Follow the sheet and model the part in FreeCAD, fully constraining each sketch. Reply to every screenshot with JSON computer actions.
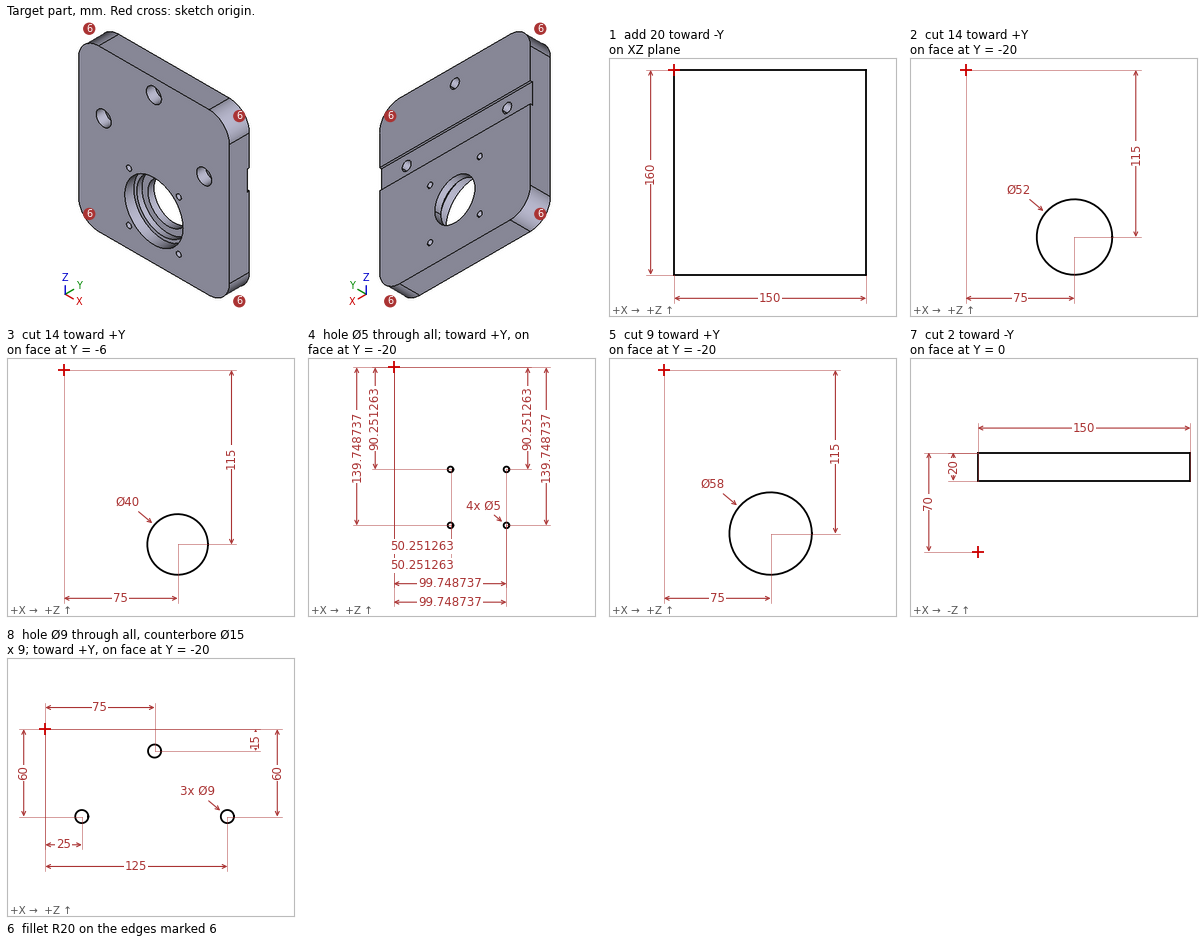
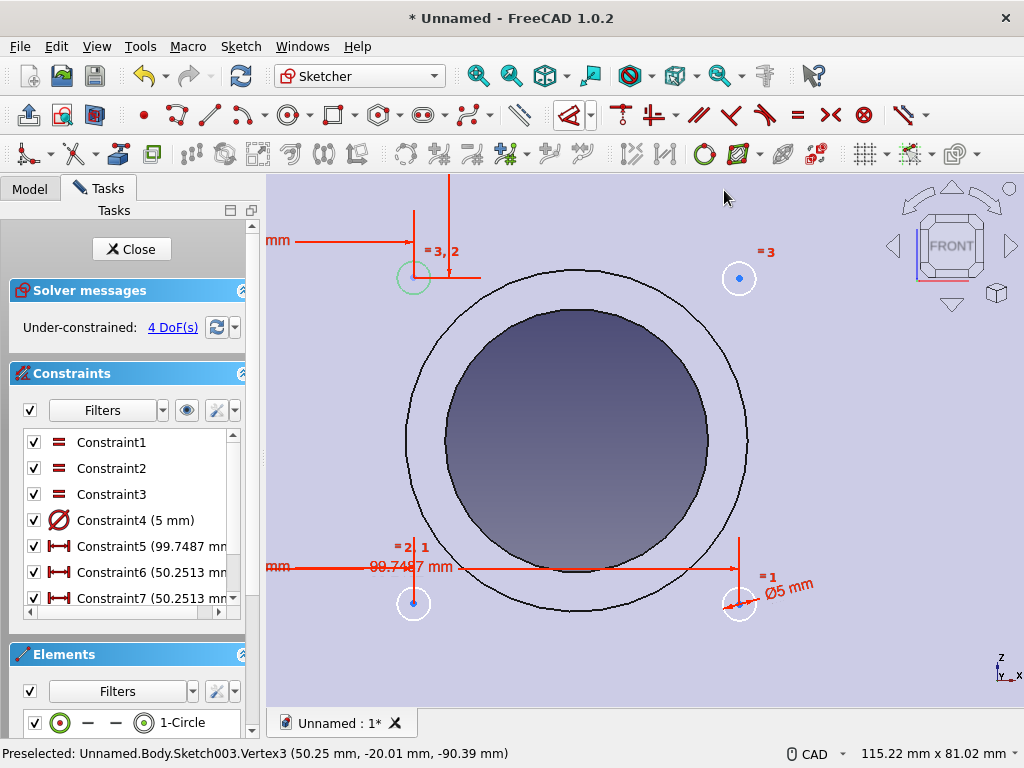
{"action": "left_click", "coordinate": [739, 279]}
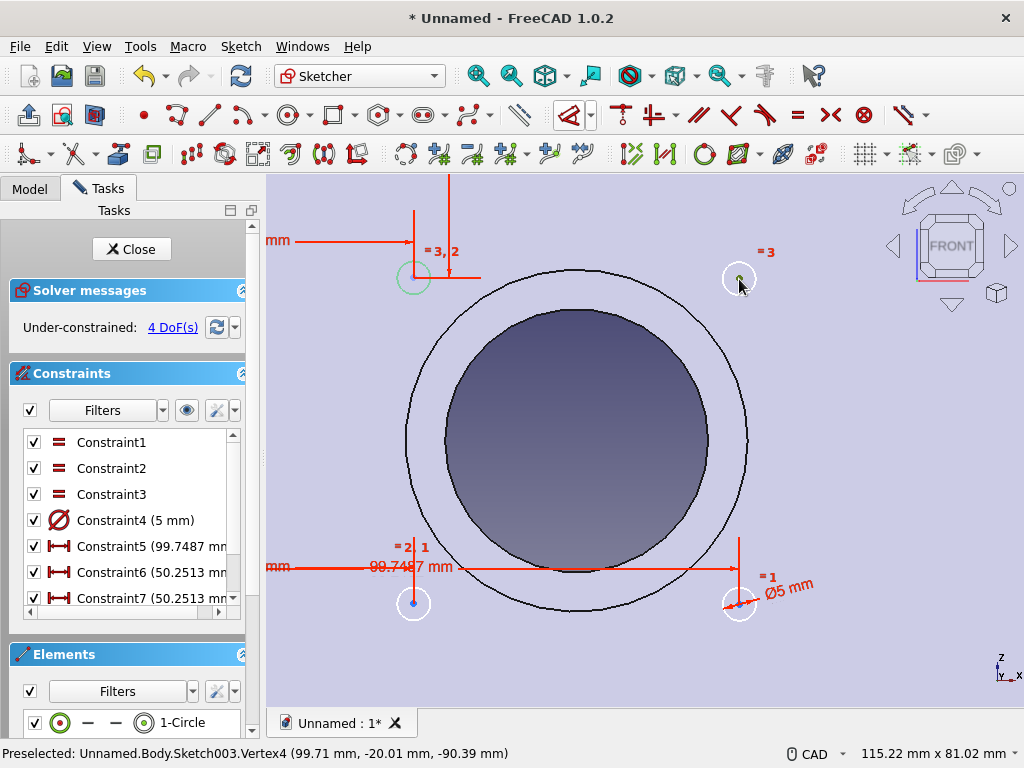
{"action": "key", "text": "l"}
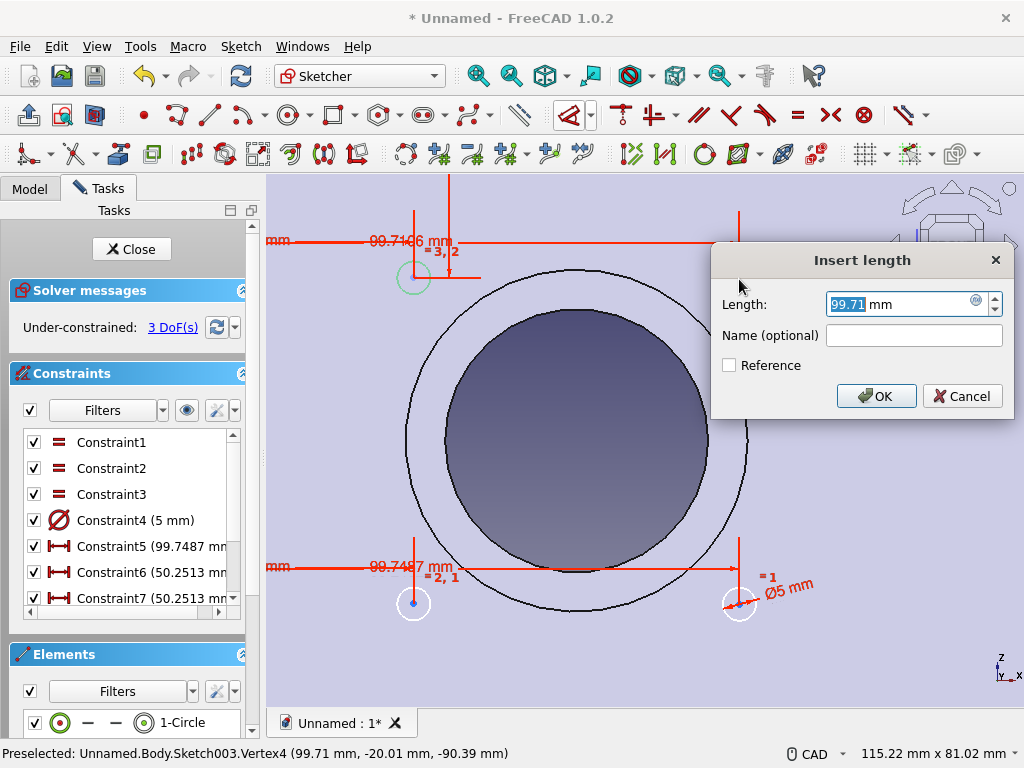
{"action": "type", "text": "99.748737"}
{"action": "key", "text": "Return"}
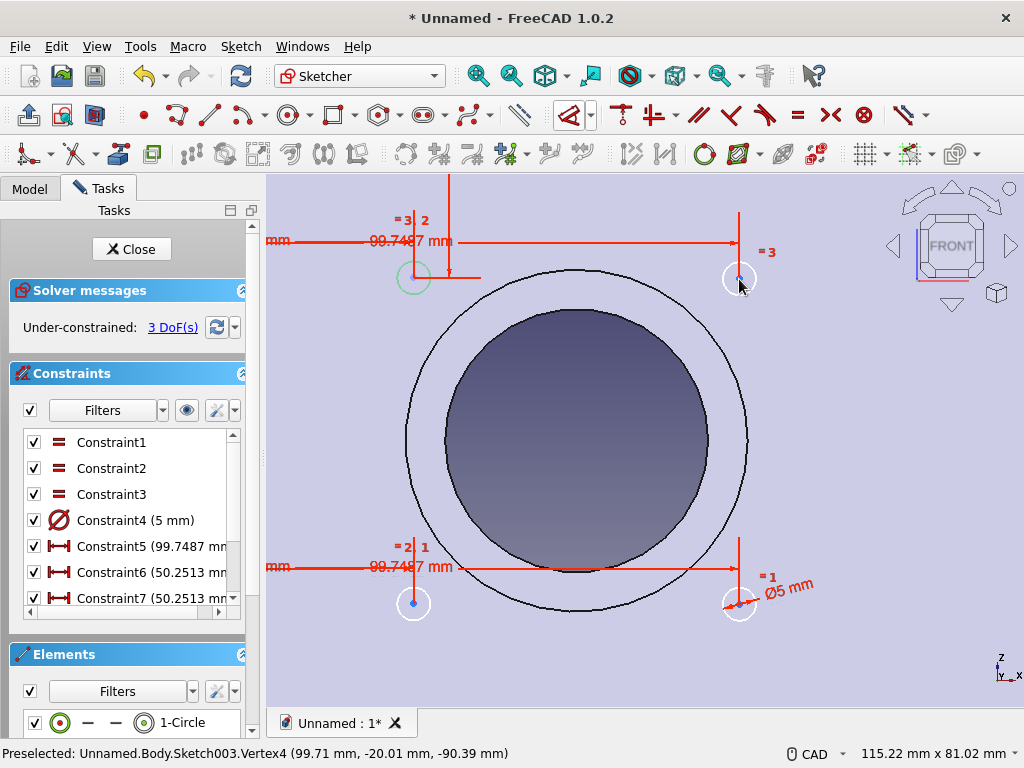
{"action": "left_click", "coordinate": [739, 279]}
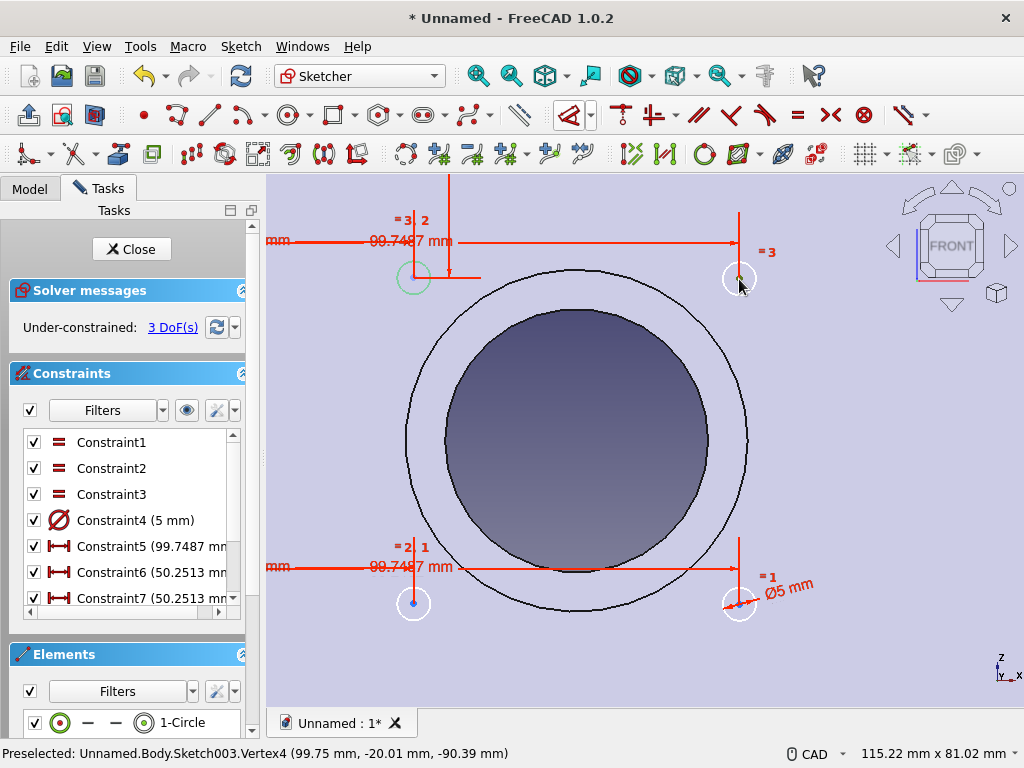
{"action": "left_click", "coordinate": [590, 116]}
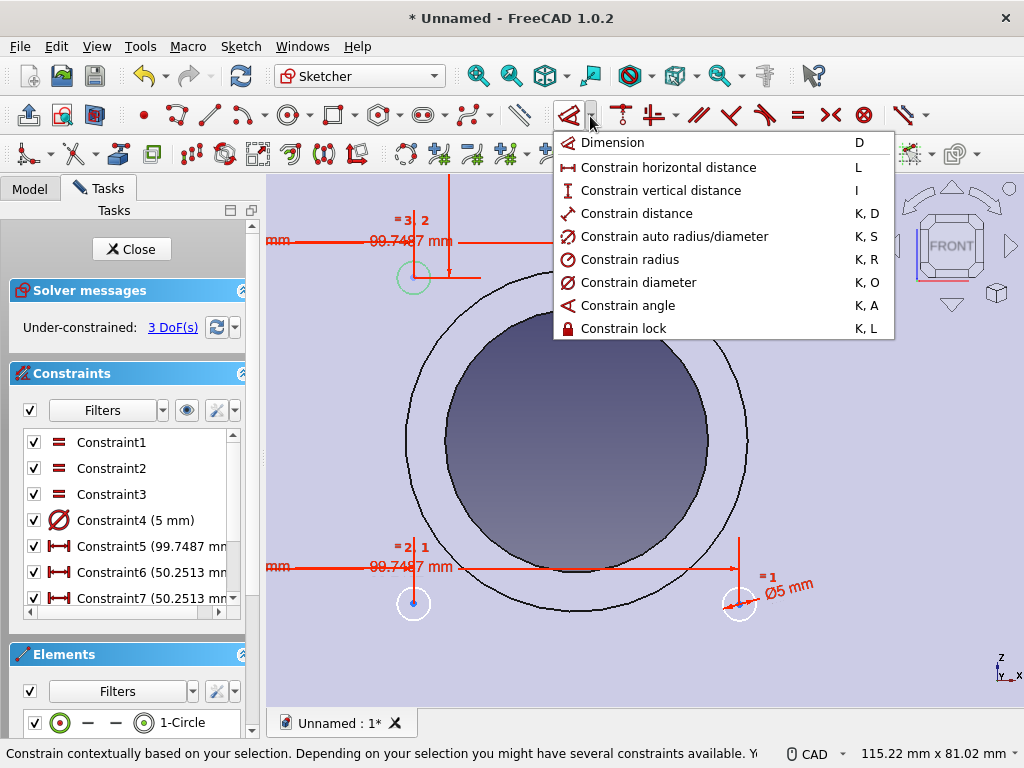
{"action": "left_click", "coordinate": [724, 190]}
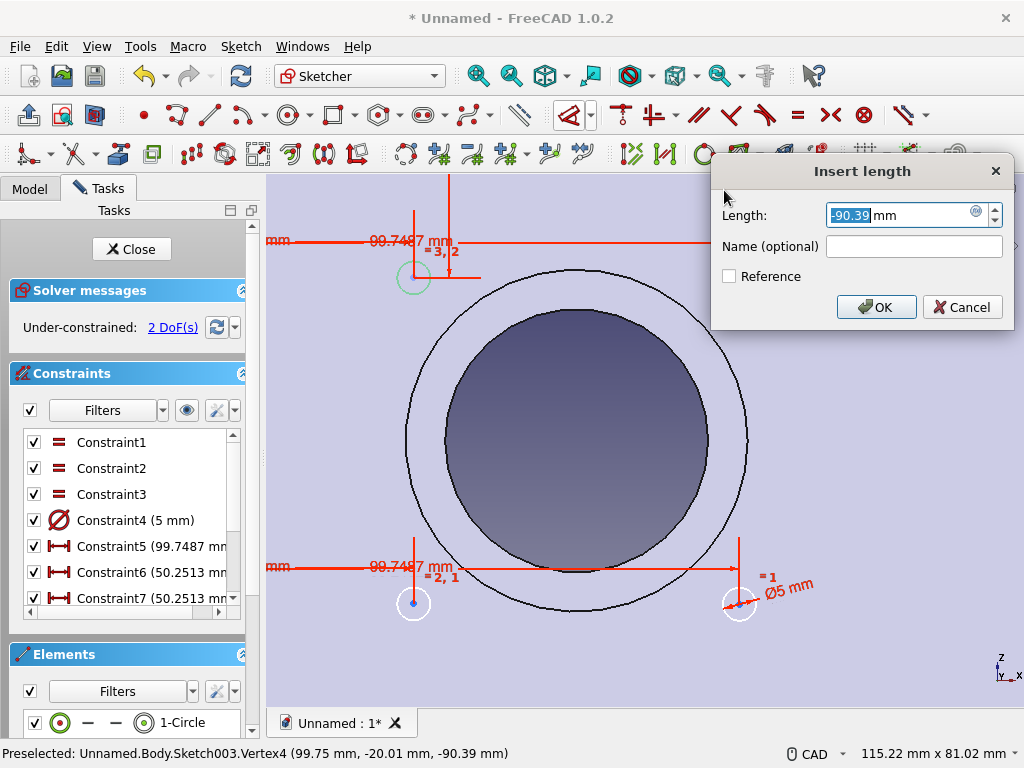
{"action": "type", "text": "-90.251263"}
{"action": "key", "text": "Return"}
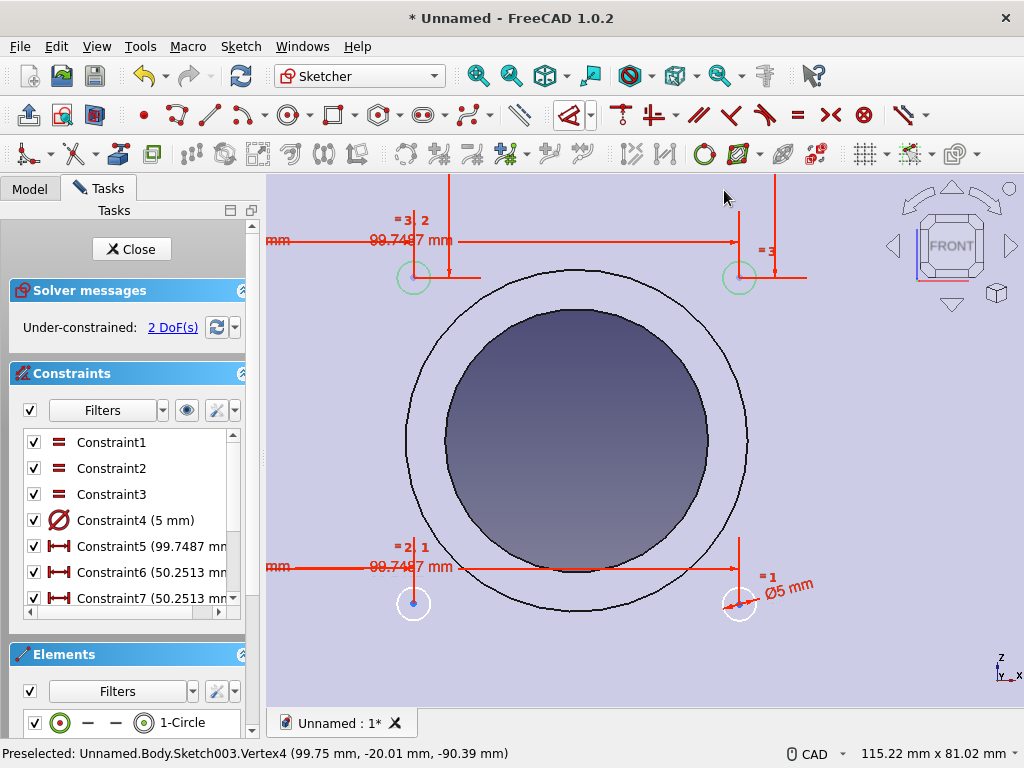
{"action": "left_click", "coordinate": [739, 604]}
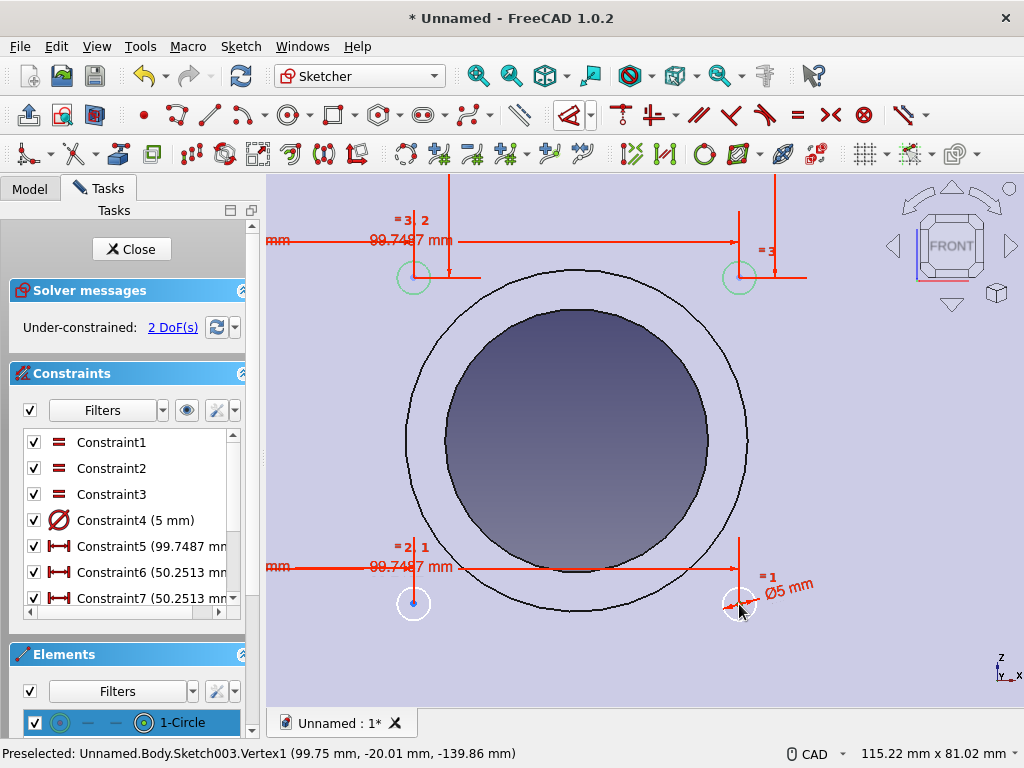
{"action": "key", "text": "i"}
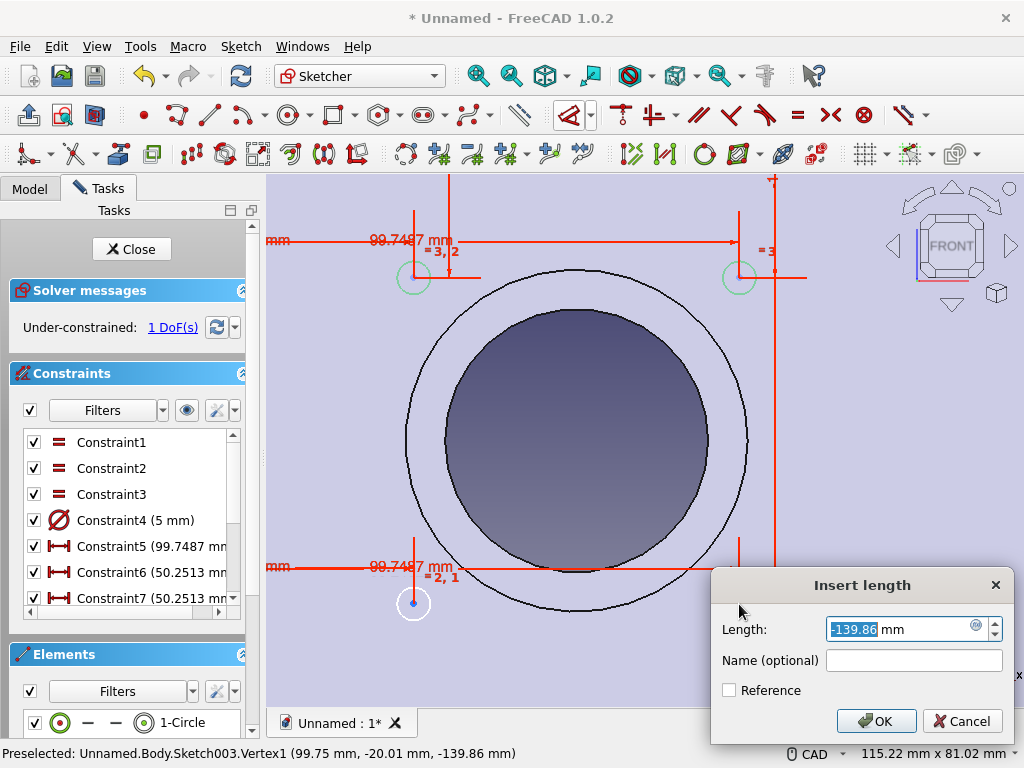
{"action": "type", "text": "-139.748737"}
{"action": "key", "text": "Return"}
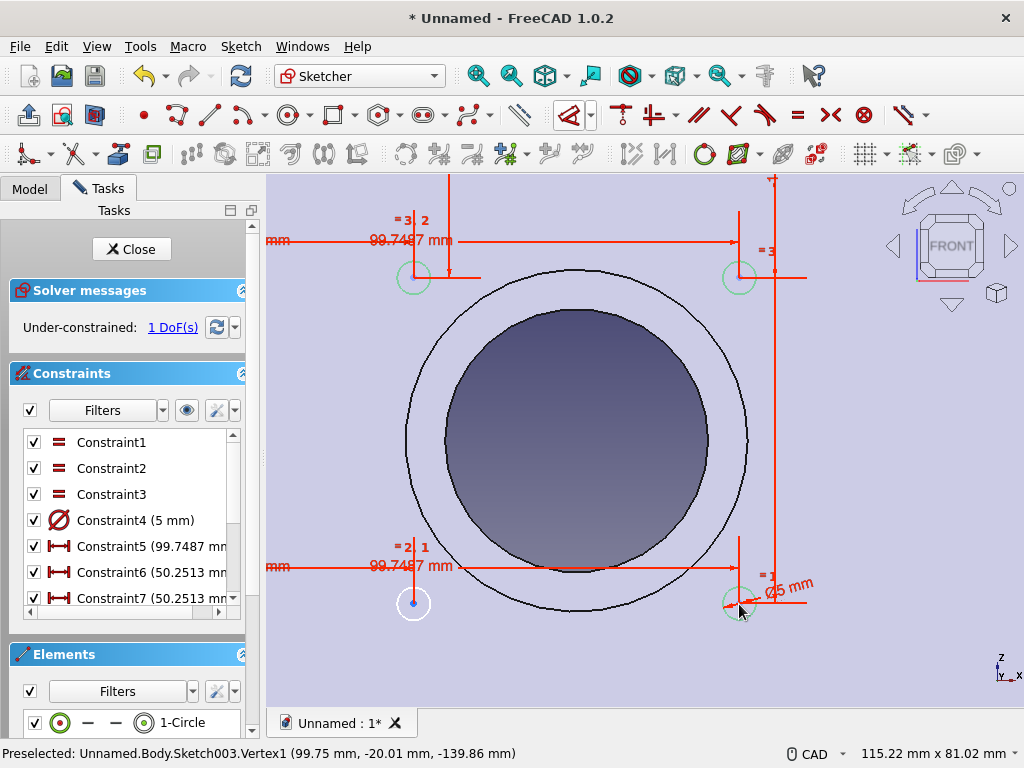
{"action": "left_click", "coordinate": [414, 604]}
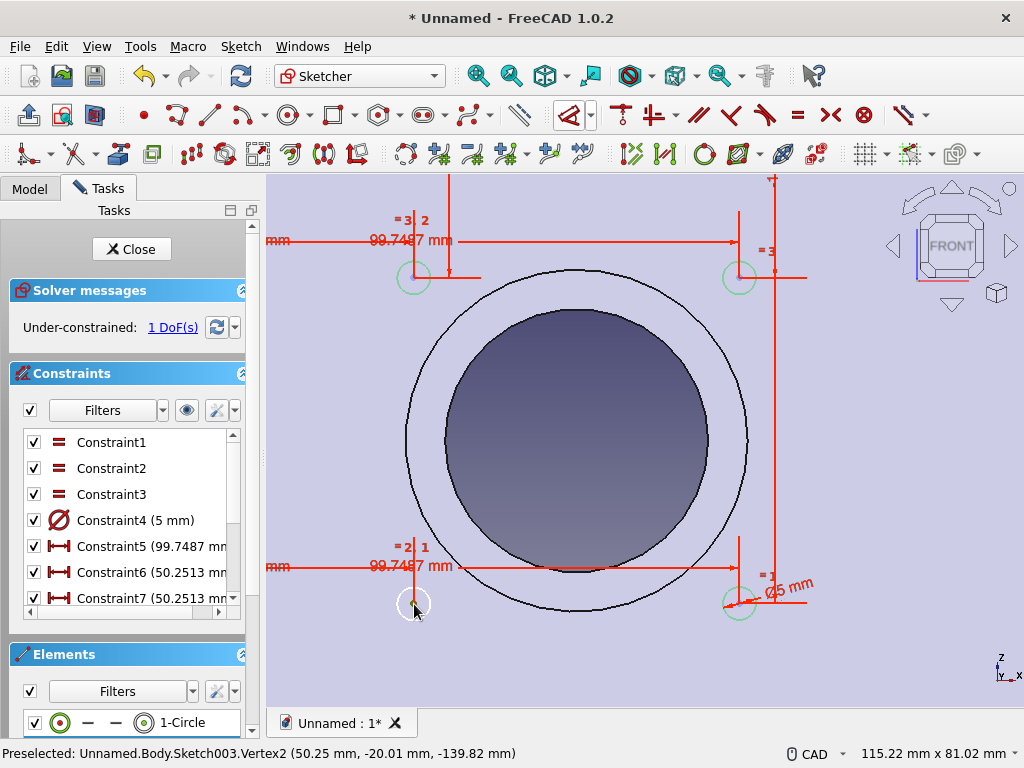
{"action": "left_click", "coordinate": [590, 116]}